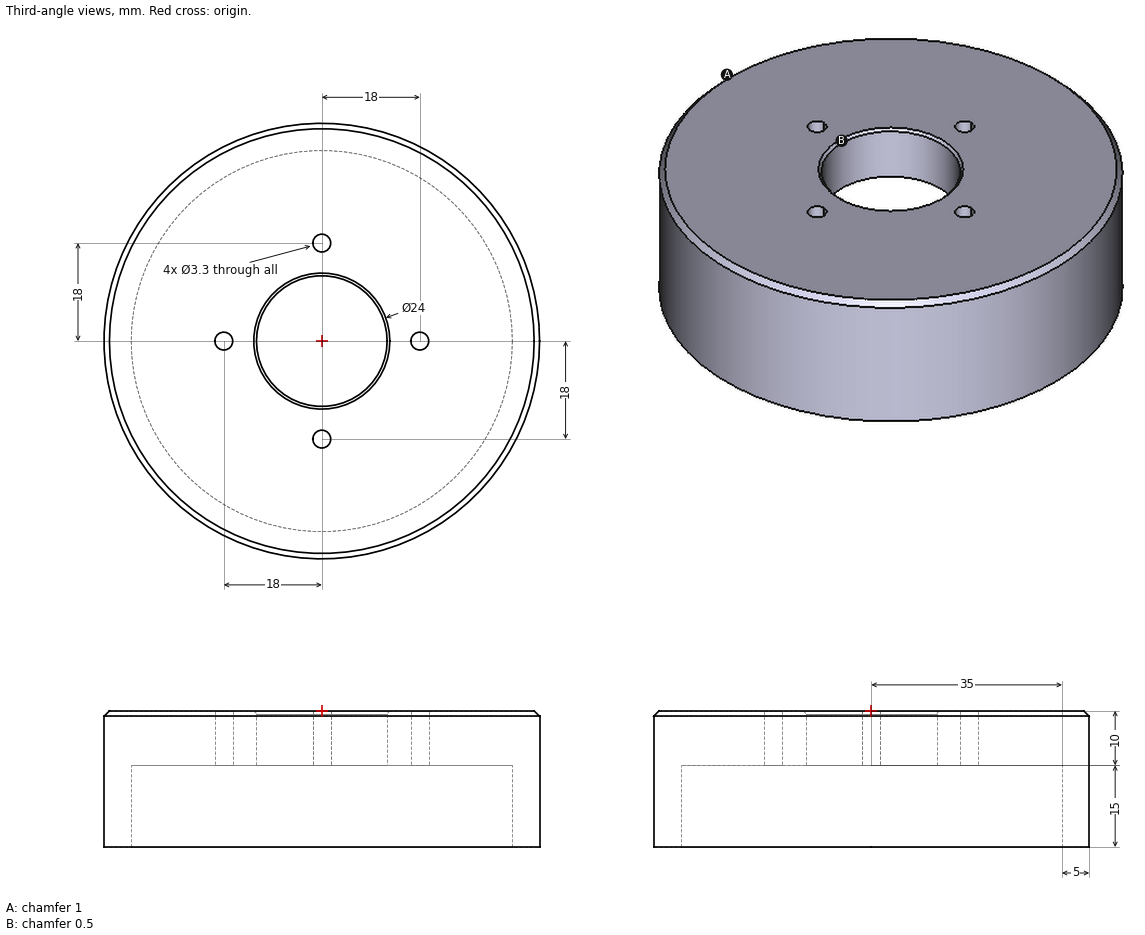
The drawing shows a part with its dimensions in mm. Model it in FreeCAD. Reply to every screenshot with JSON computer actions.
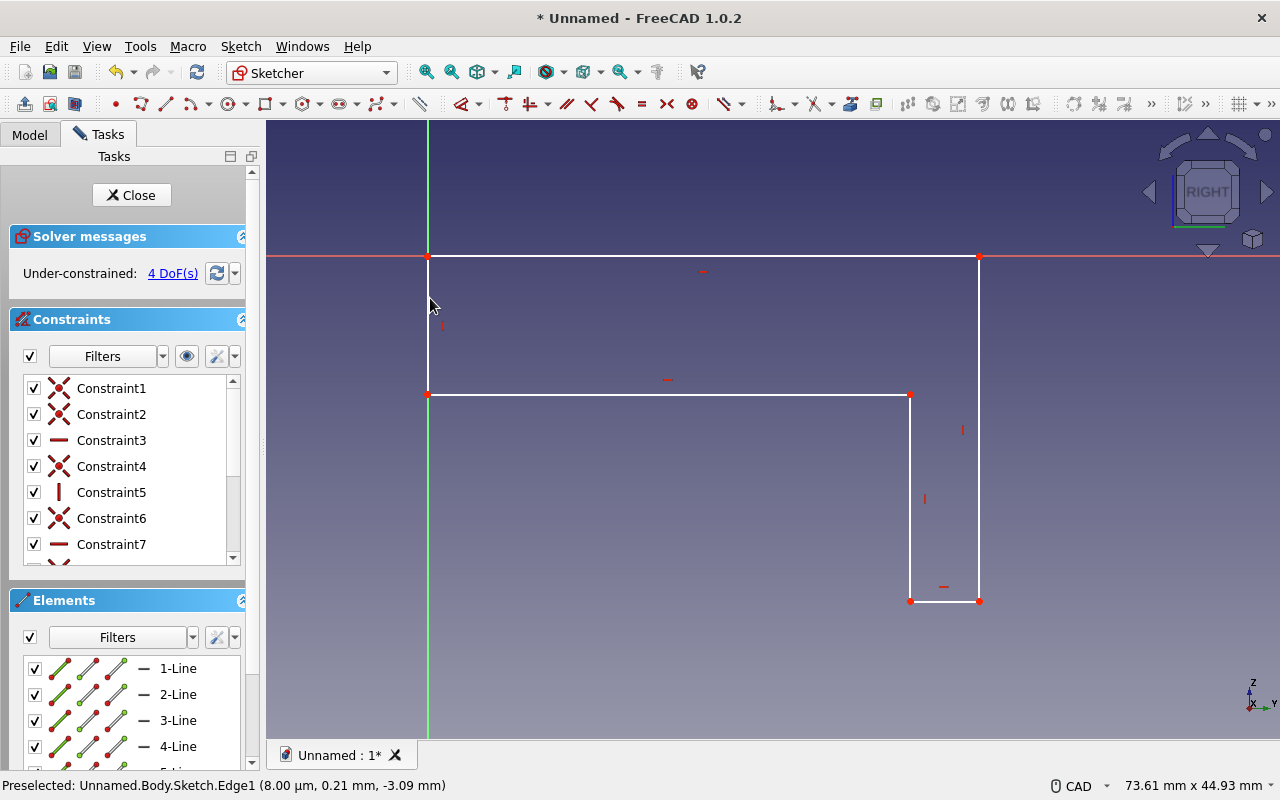
{"action": "left_click", "coordinate": [460, 104]}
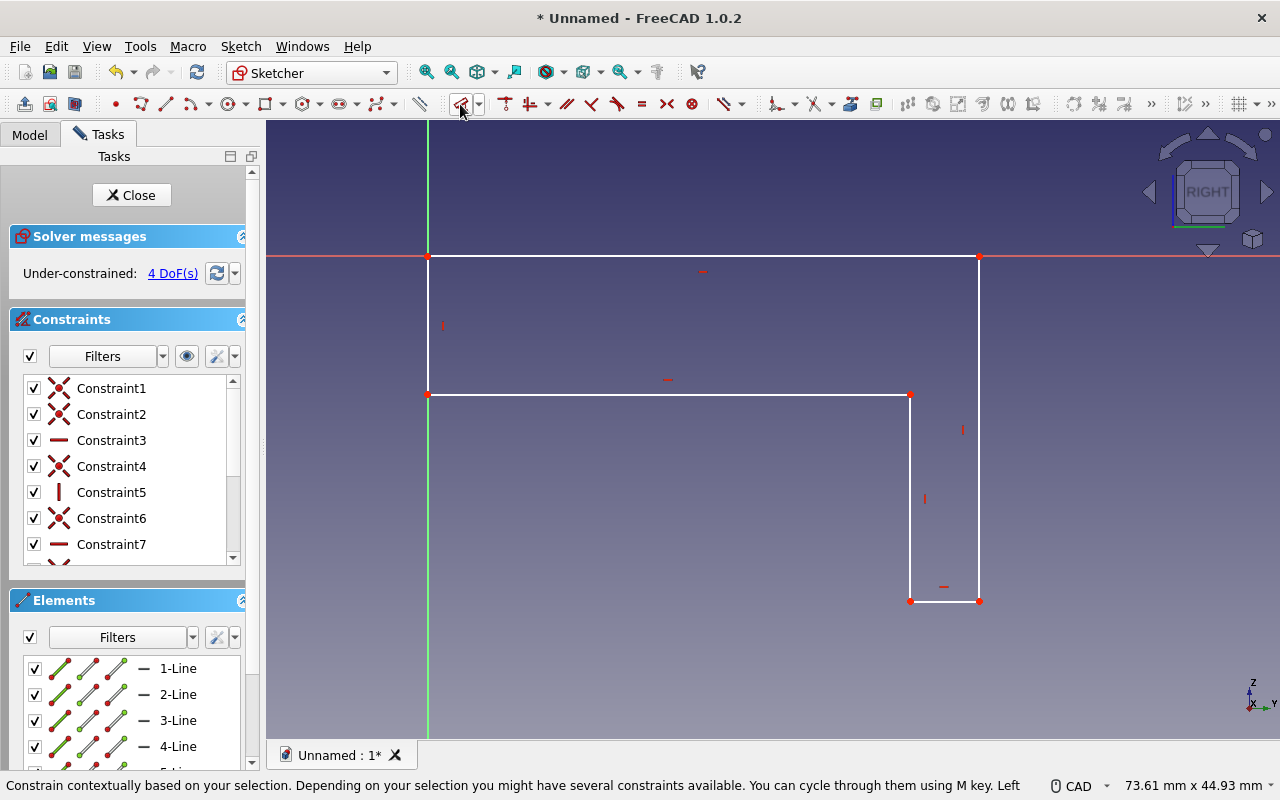
{"action": "left_click", "coordinate": [931, 602]}
{"action": "left_click", "coordinate": [944, 636]}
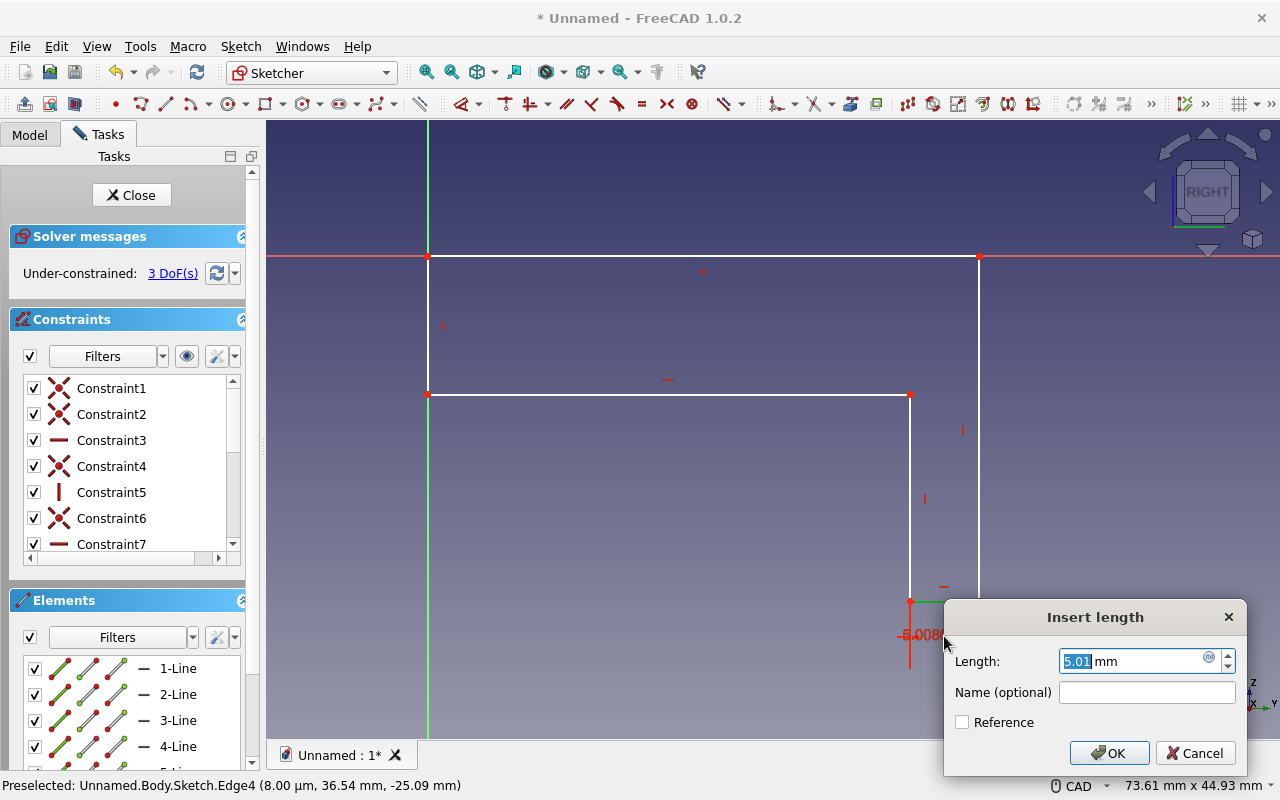
{"action": "type", "text": "5"}
{"action": "key", "text": "Return"}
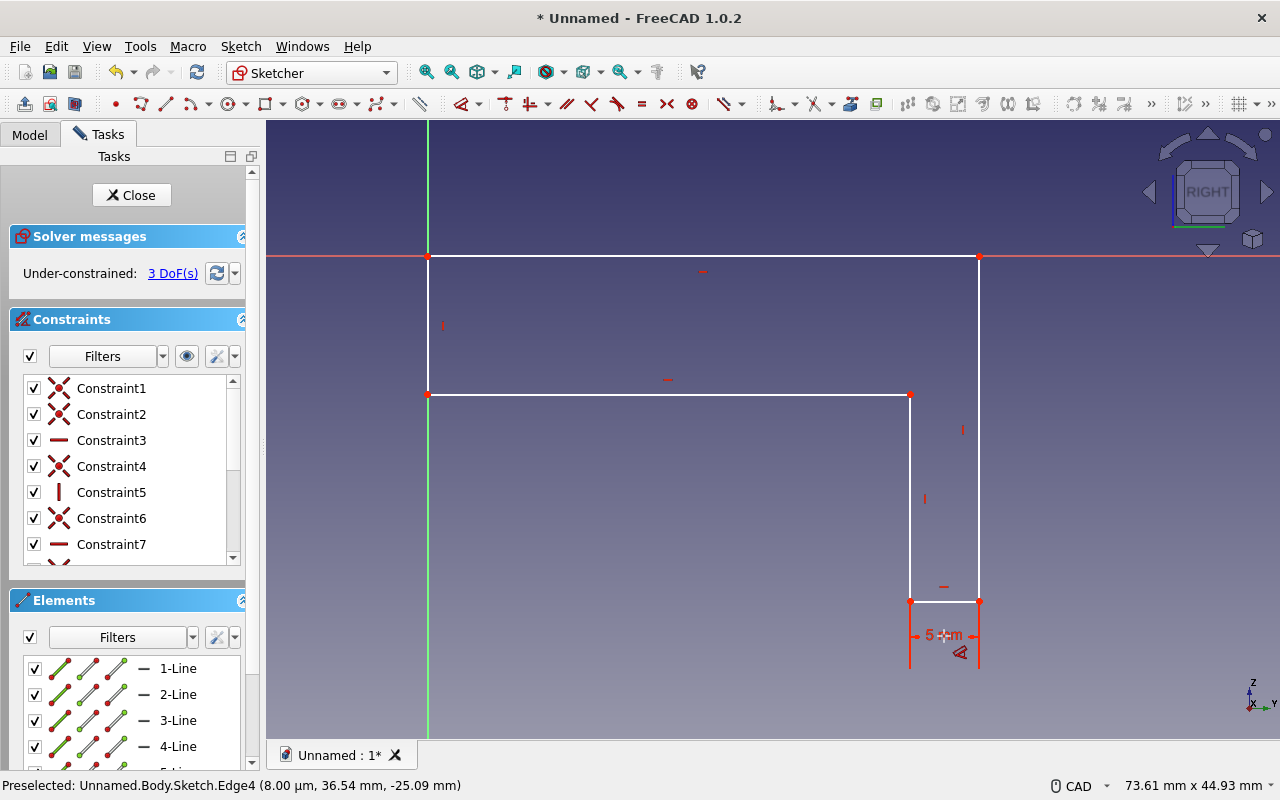
{"action": "left_click", "coordinate": [428, 298]}
{"action": "left_click", "coordinate": [394, 326]}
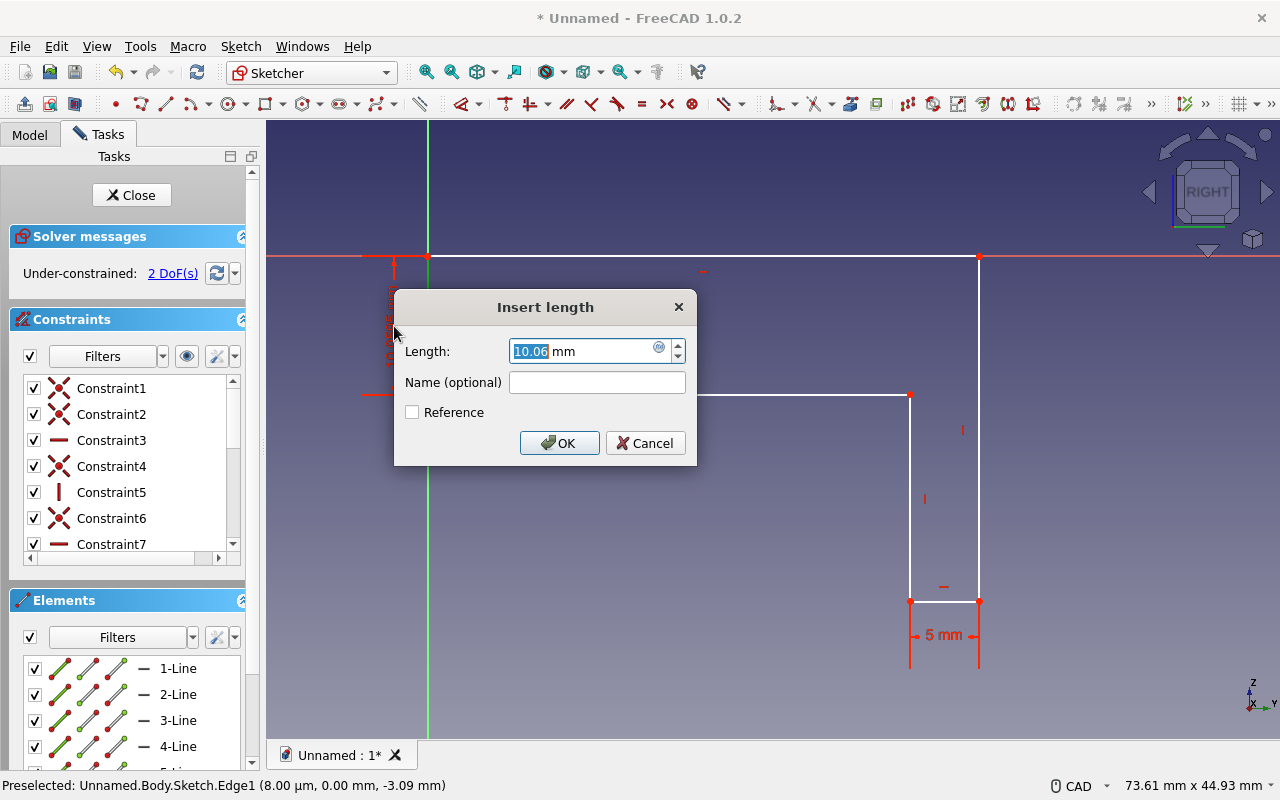
{"action": "type", "text": "10"}
{"action": "key", "text": "Return"}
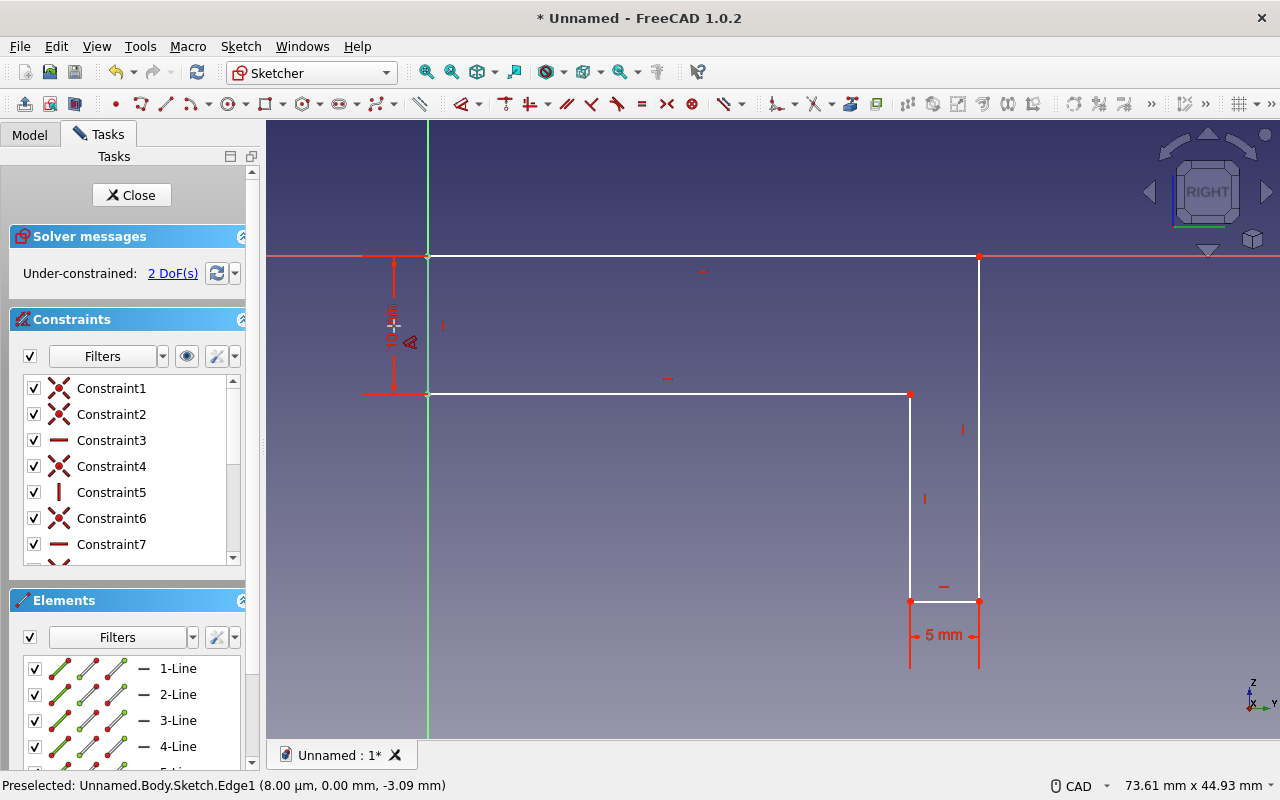
{"action": "left_click", "coordinate": [572, 394]}
{"action": "left_click", "coordinate": [669, 360]}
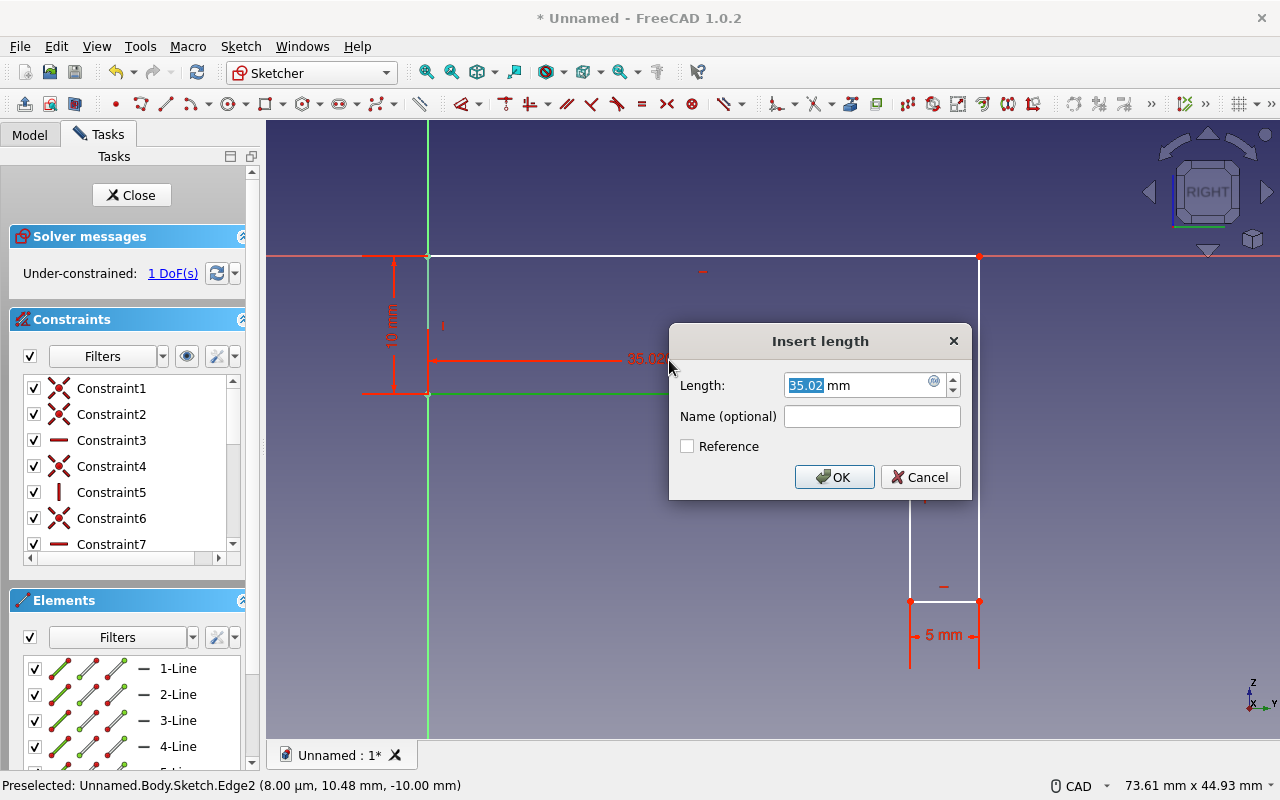
{"action": "type", "text": "35"}
{"action": "key", "text": "Return"}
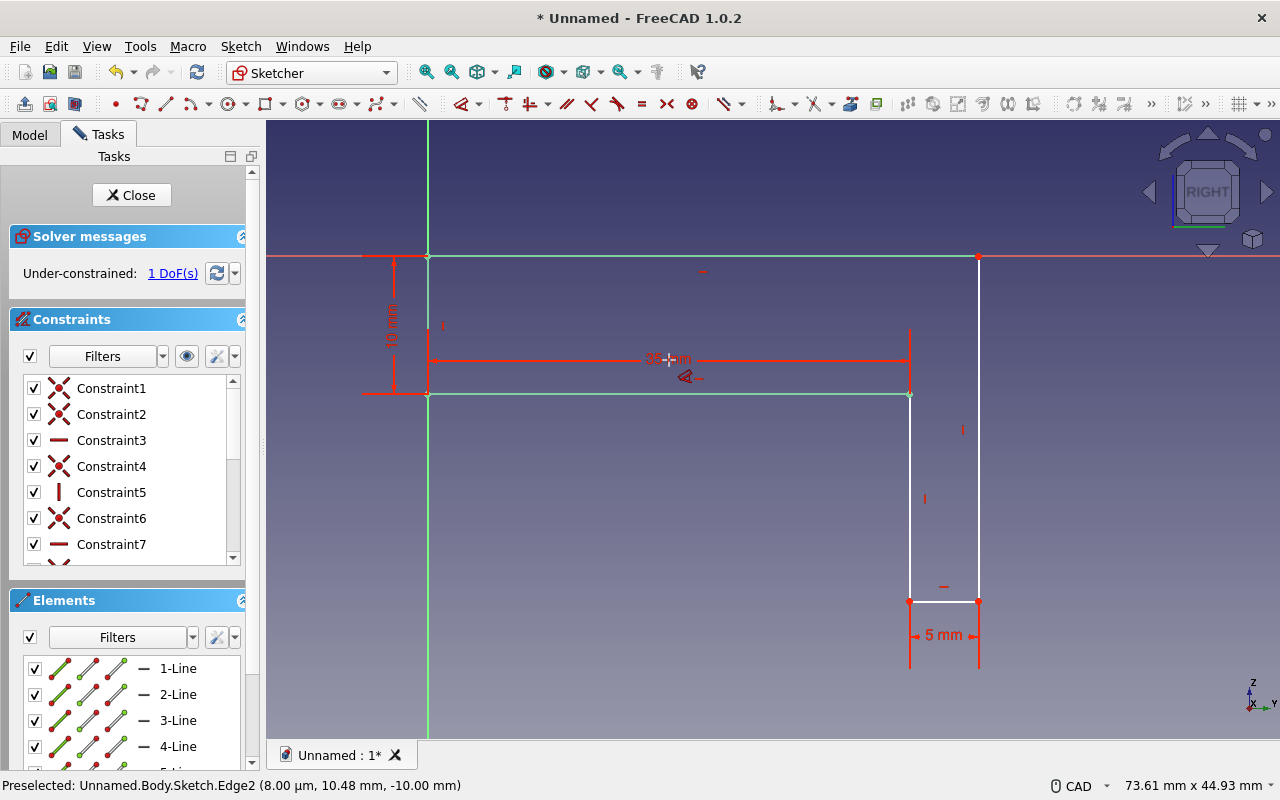
{"action": "left_click", "coordinate": [910, 457]}
{"action": "left_click", "coordinate": [944, 498]}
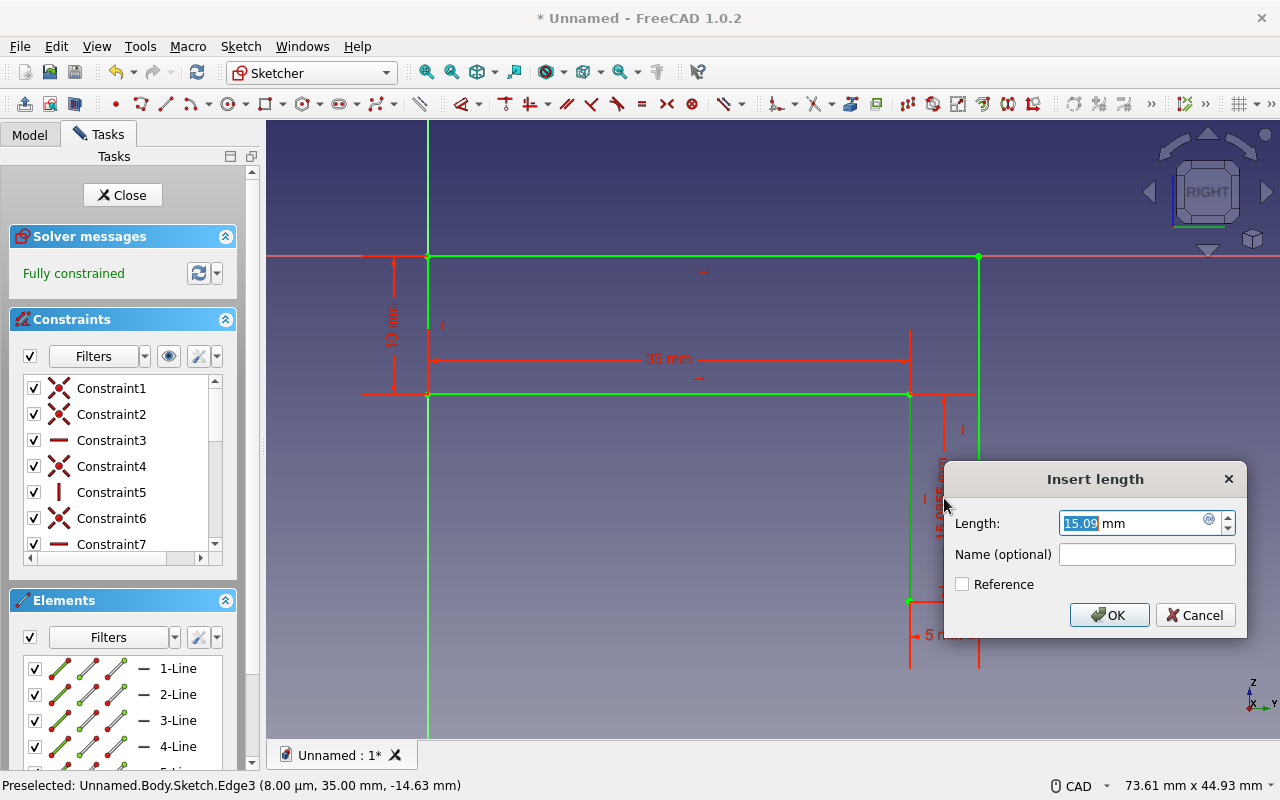
{"action": "type", "text": "15"}
{"action": "key", "text": "Return"}
{"action": "key", "text": "Escape"}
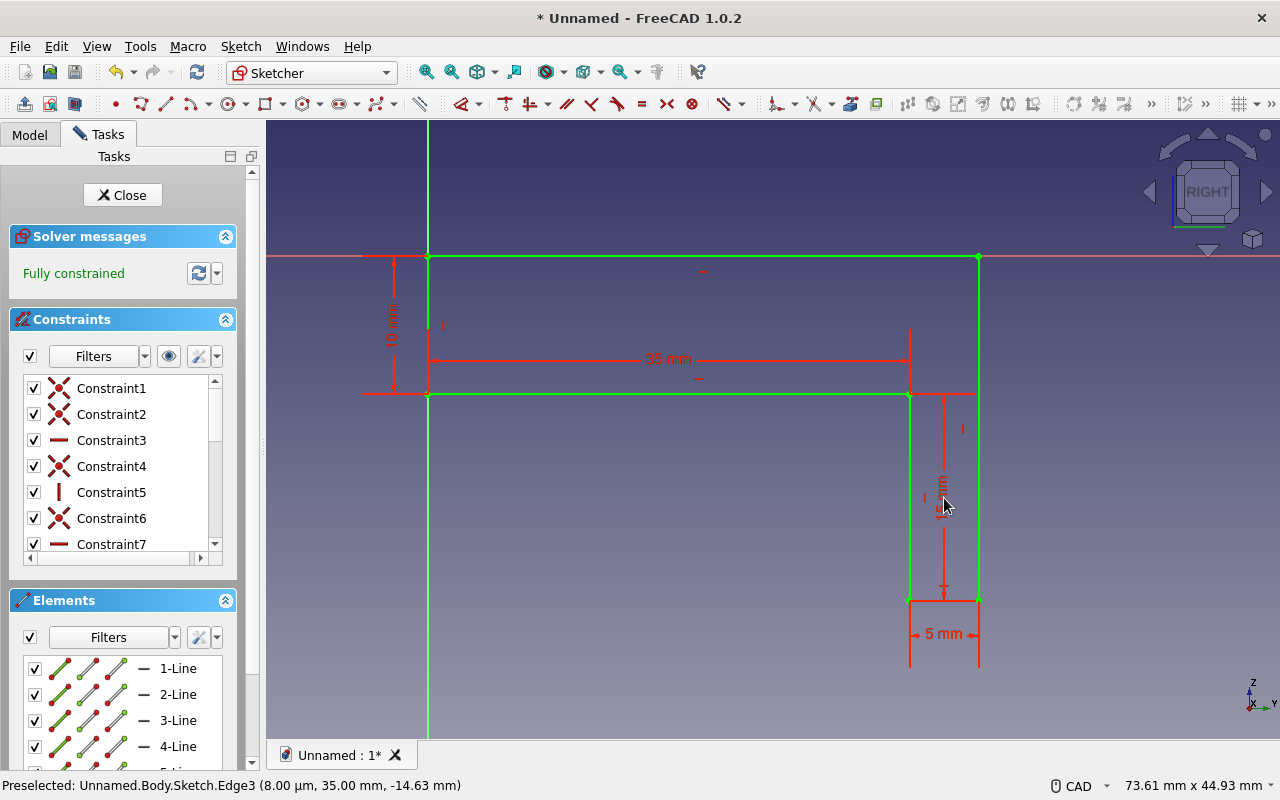
{"action": "left_click", "coordinate": [123, 195]}